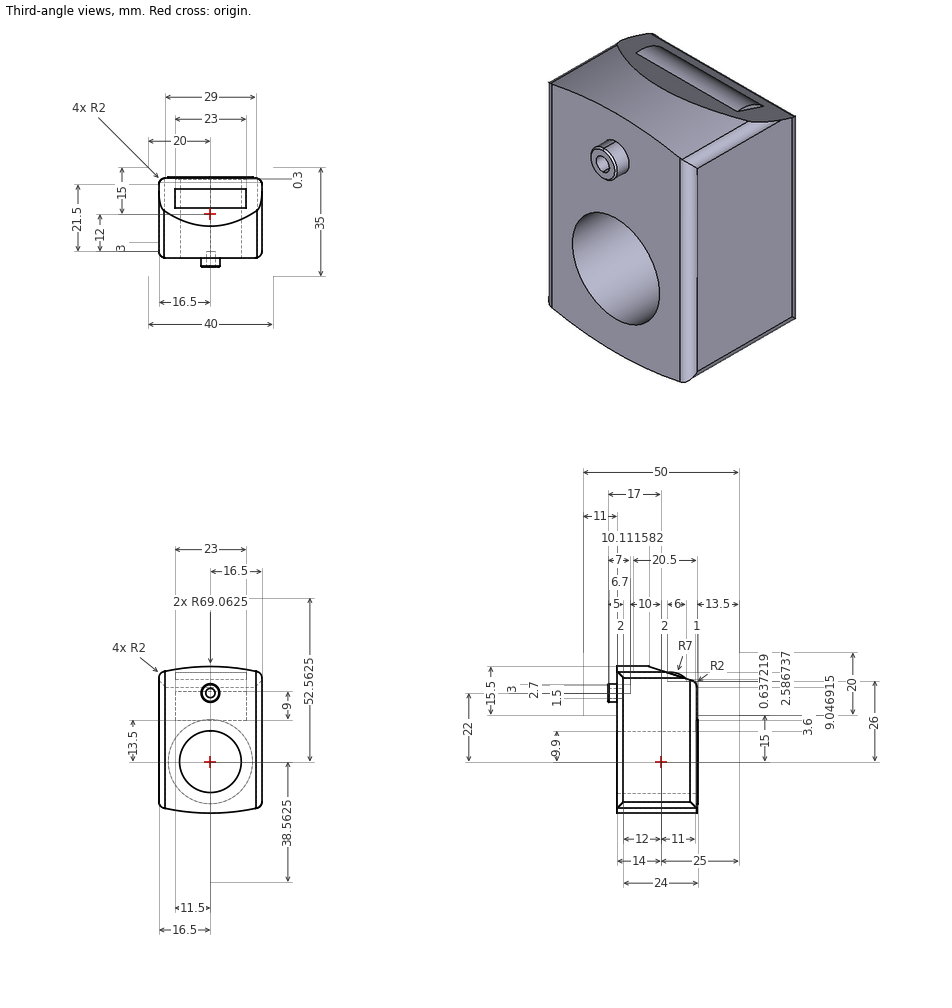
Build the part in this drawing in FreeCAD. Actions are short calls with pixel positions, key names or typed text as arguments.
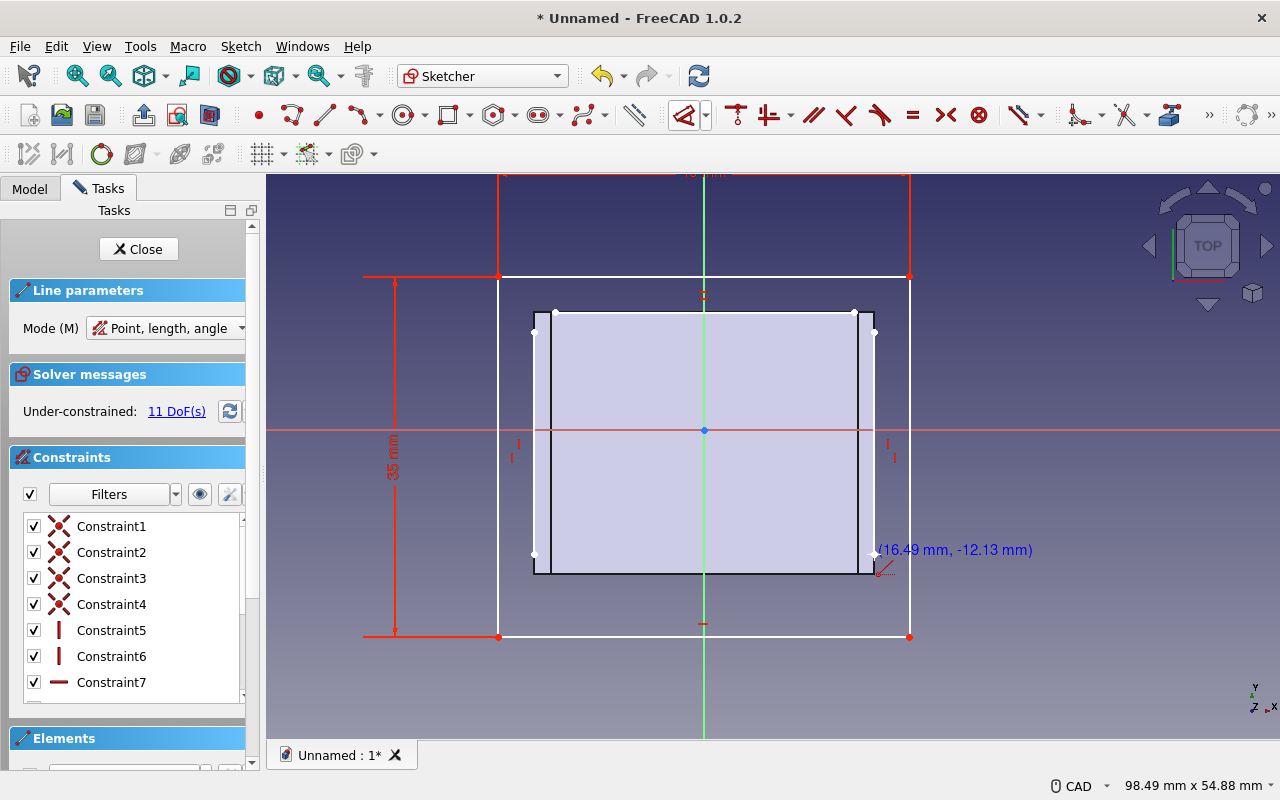
click(854, 574)
click(555, 574)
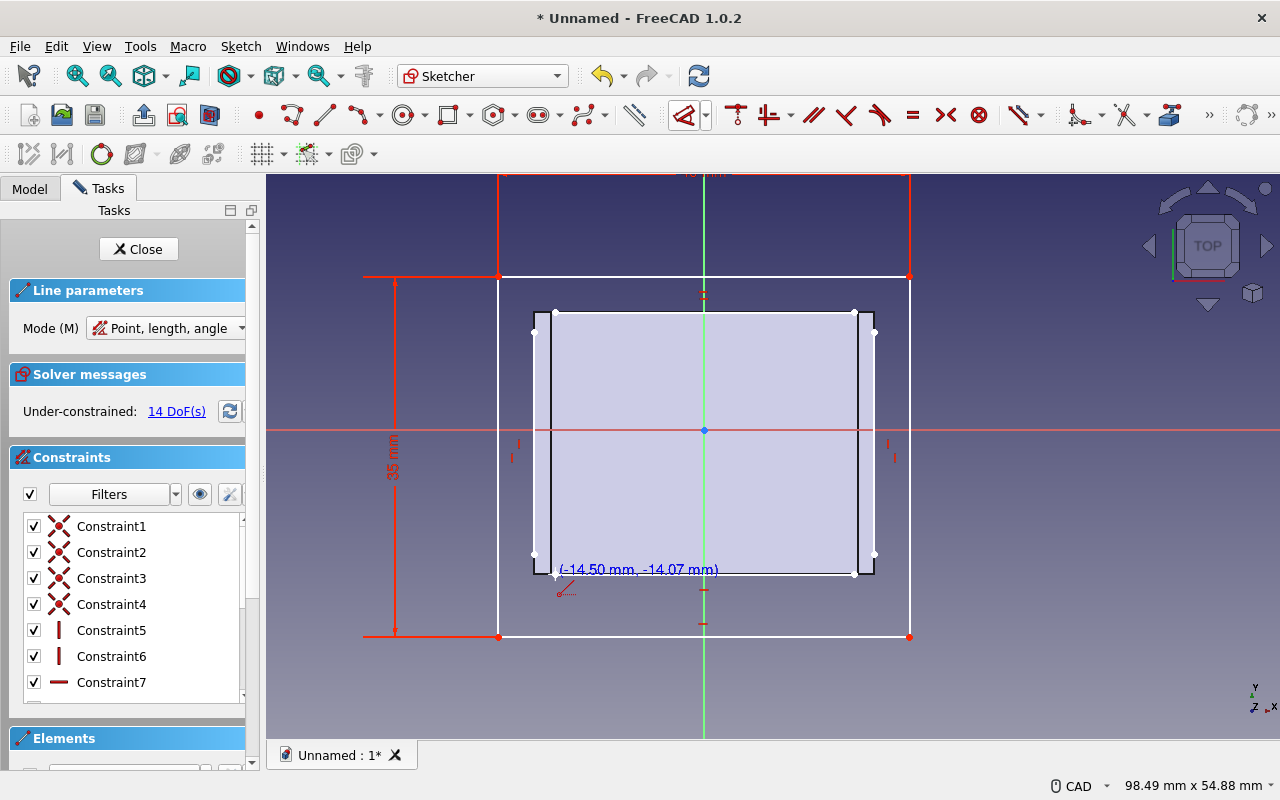
click(358, 116)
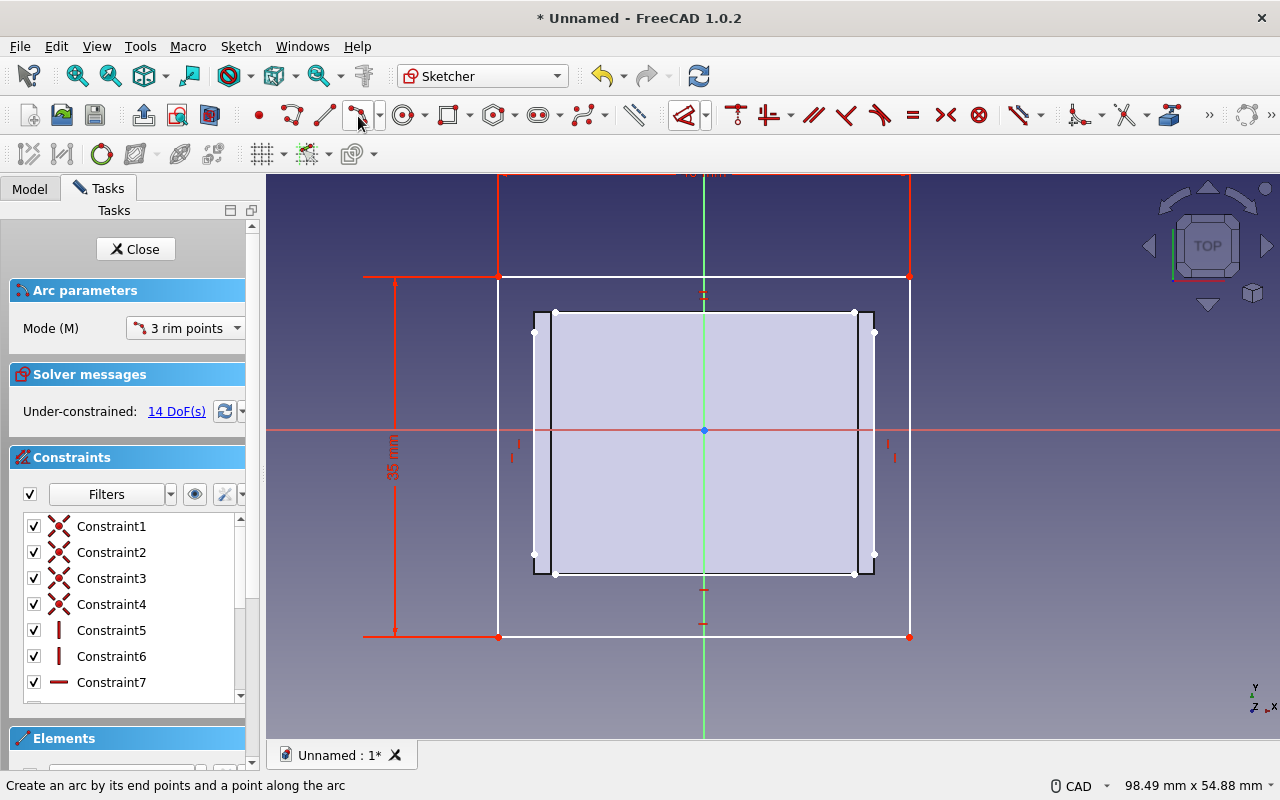
click(534, 333)
click(555, 313)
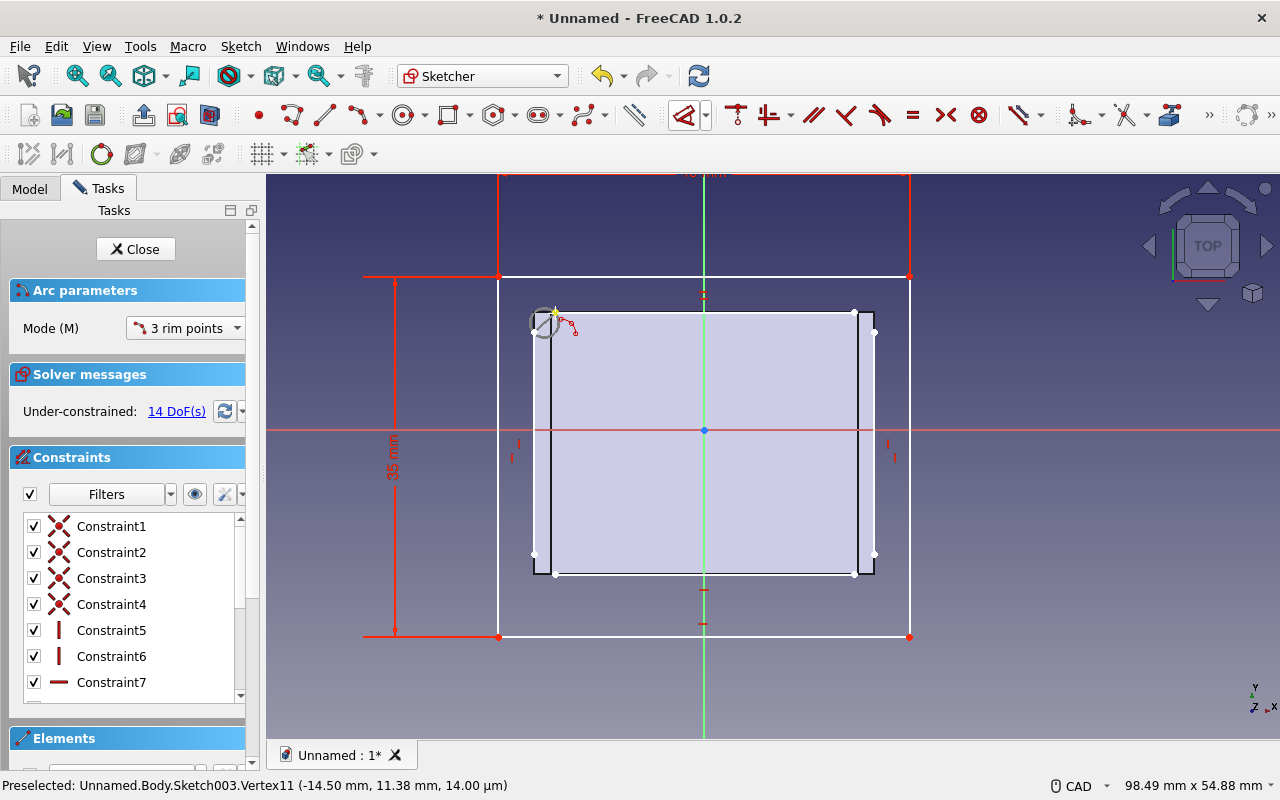
scroll(540, 318, up, 5)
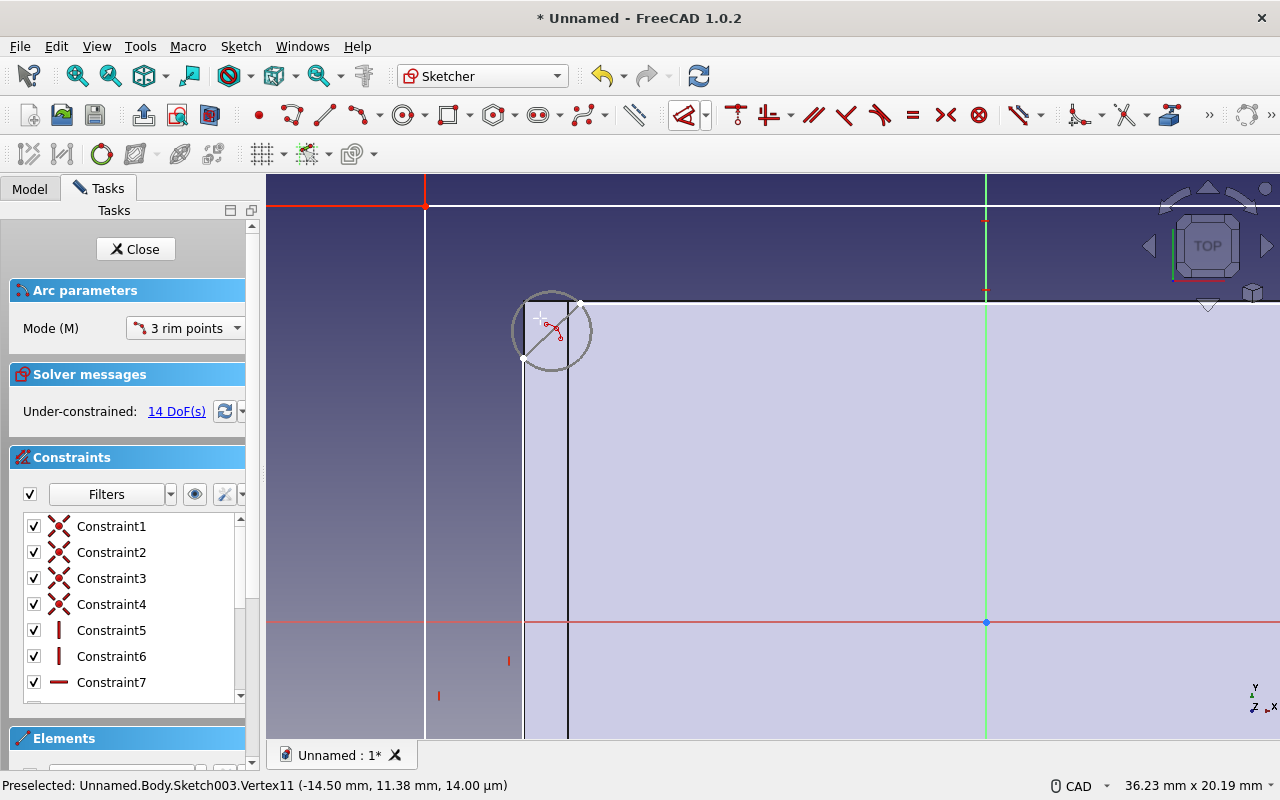
click(541, 317)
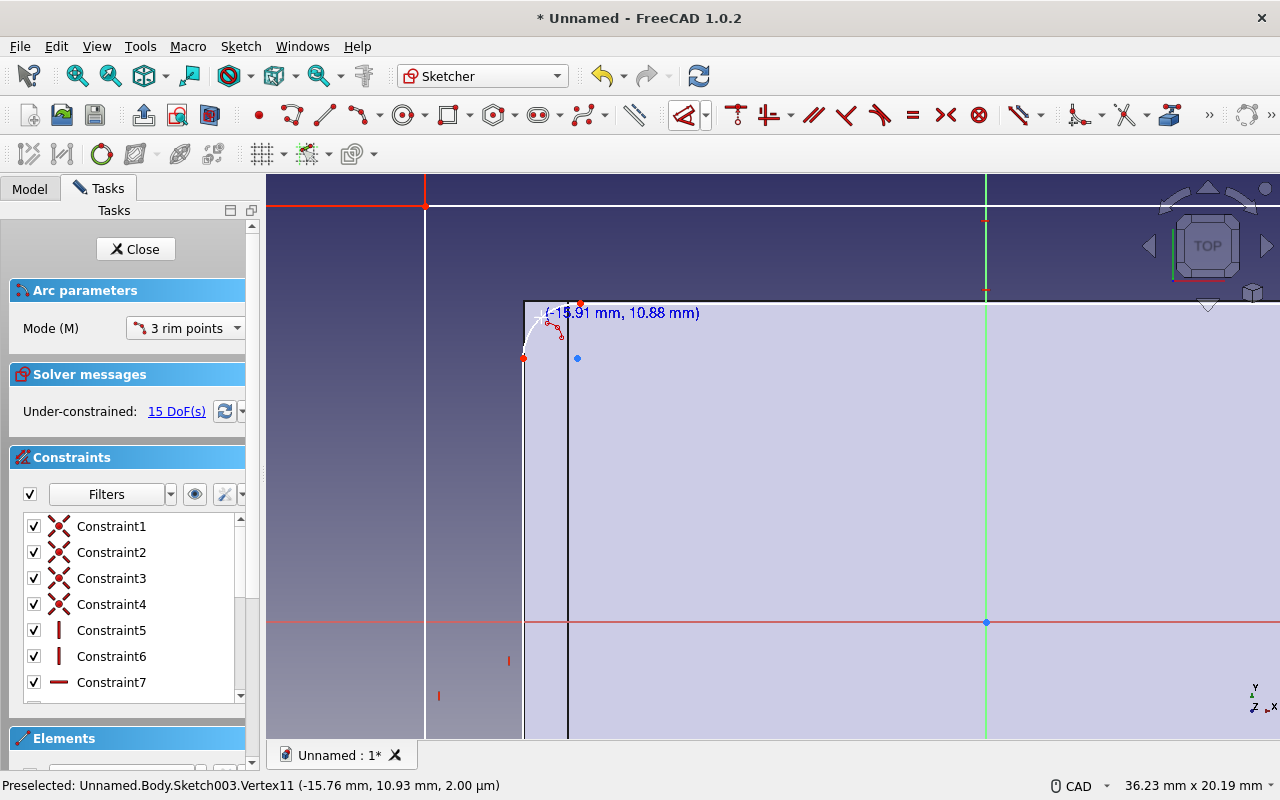
scroll(541, 319, down, 5)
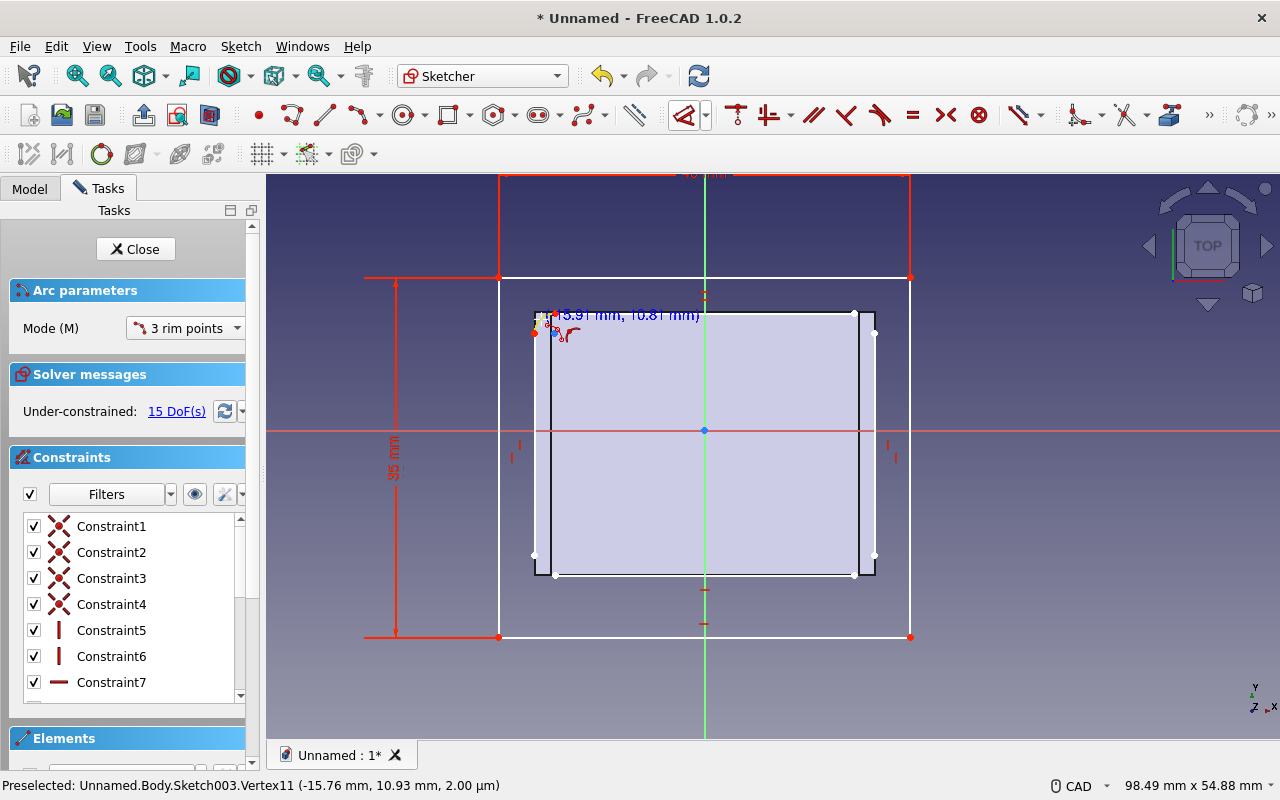
click(855, 314)
click(875, 334)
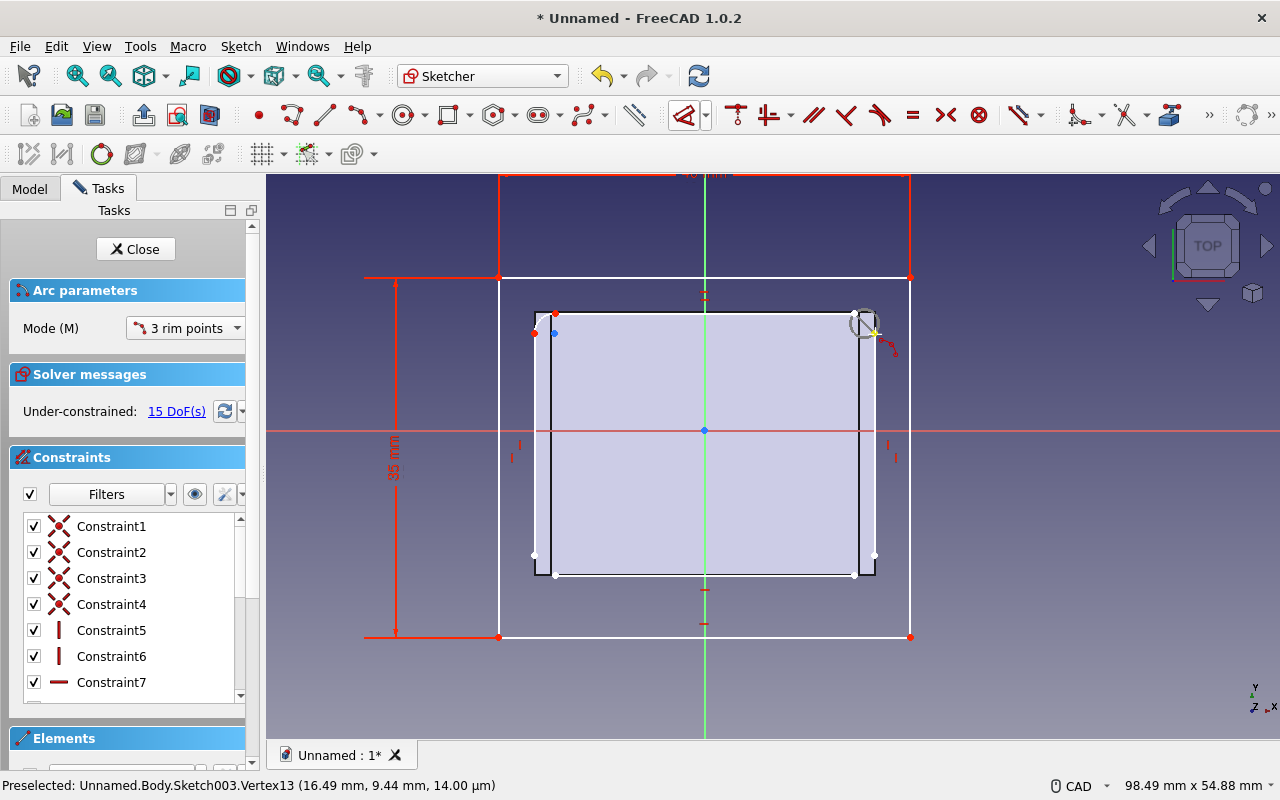
scroll(869, 318, up, 5)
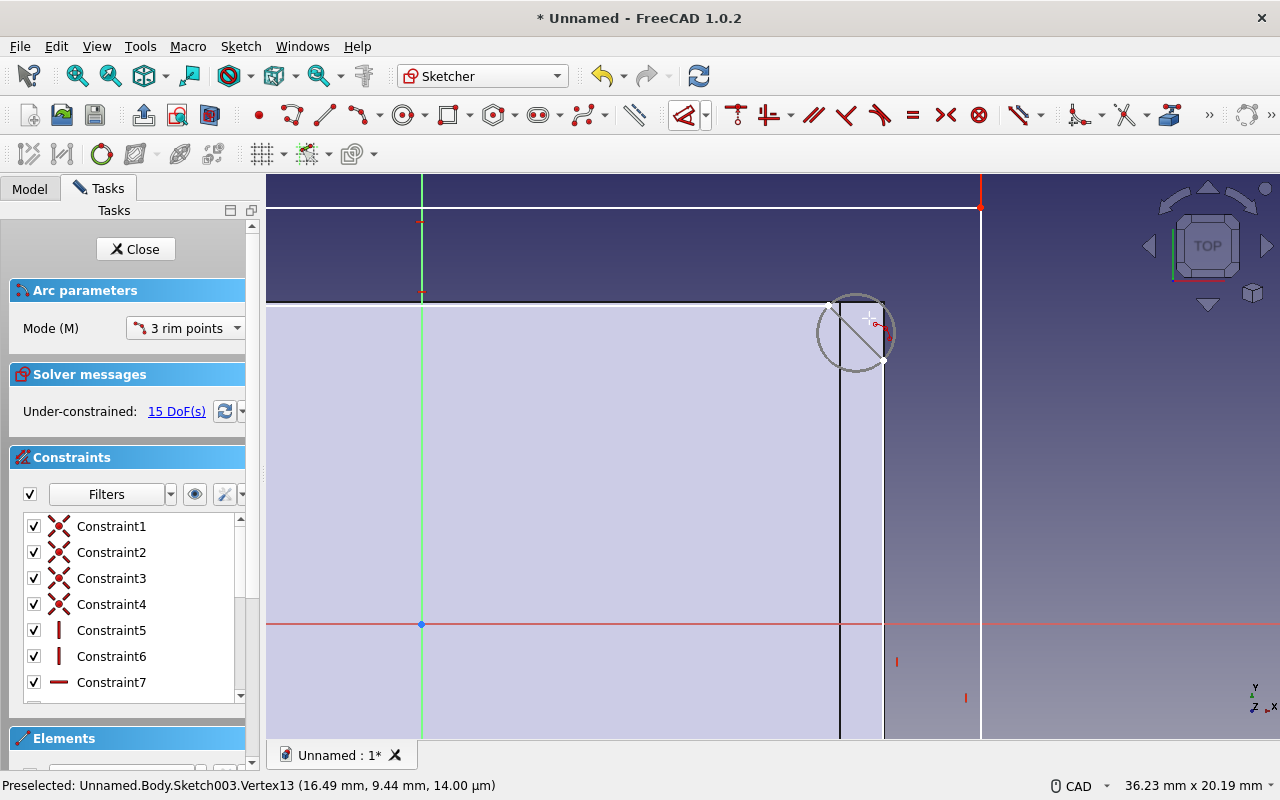
click(867, 319)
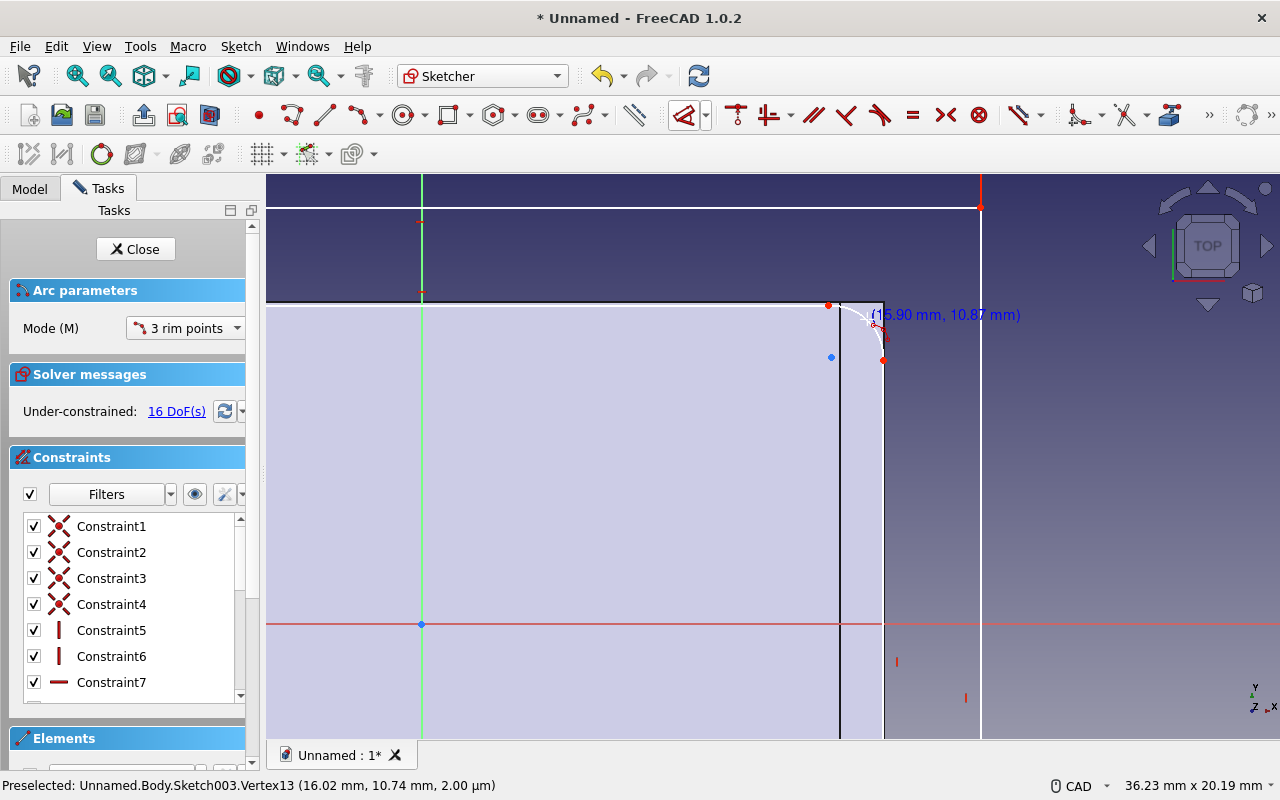
scroll(869, 318, down, 5)